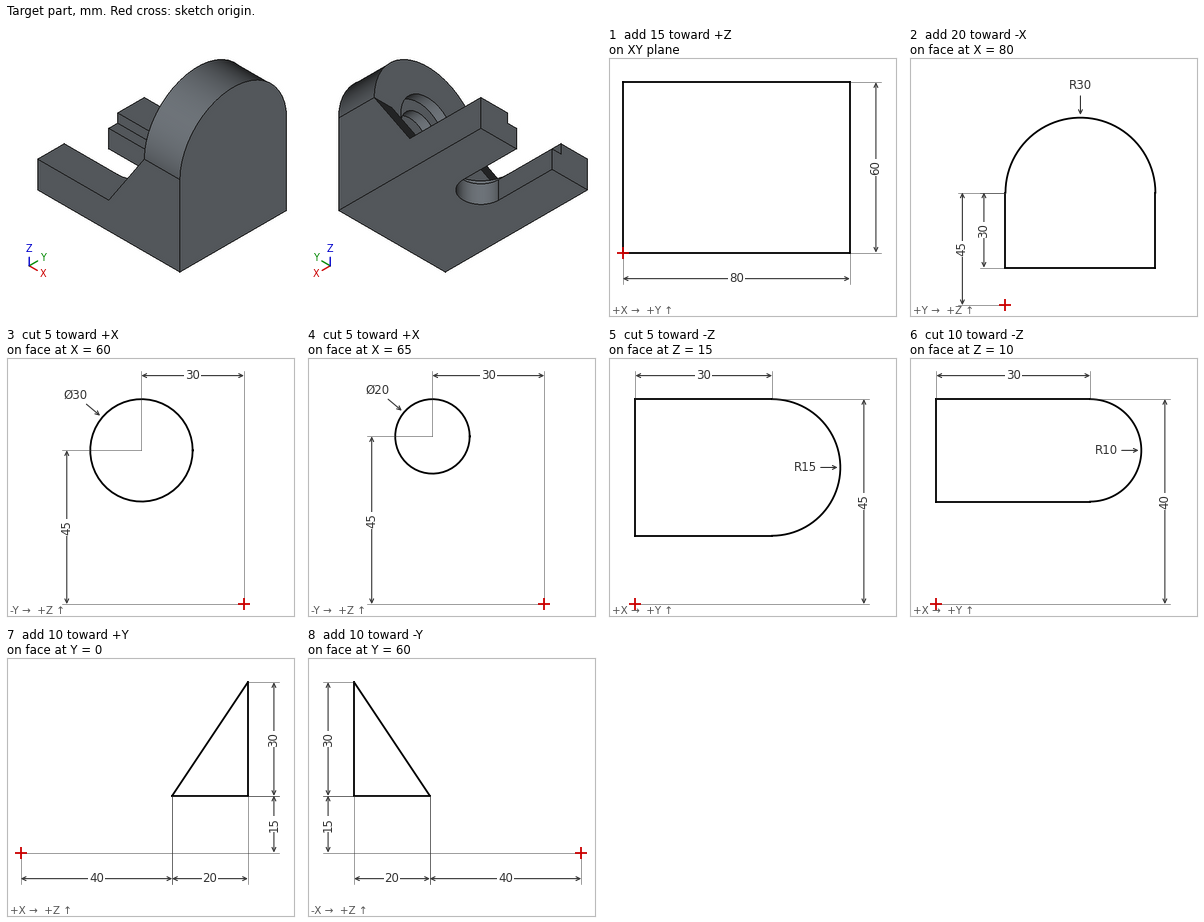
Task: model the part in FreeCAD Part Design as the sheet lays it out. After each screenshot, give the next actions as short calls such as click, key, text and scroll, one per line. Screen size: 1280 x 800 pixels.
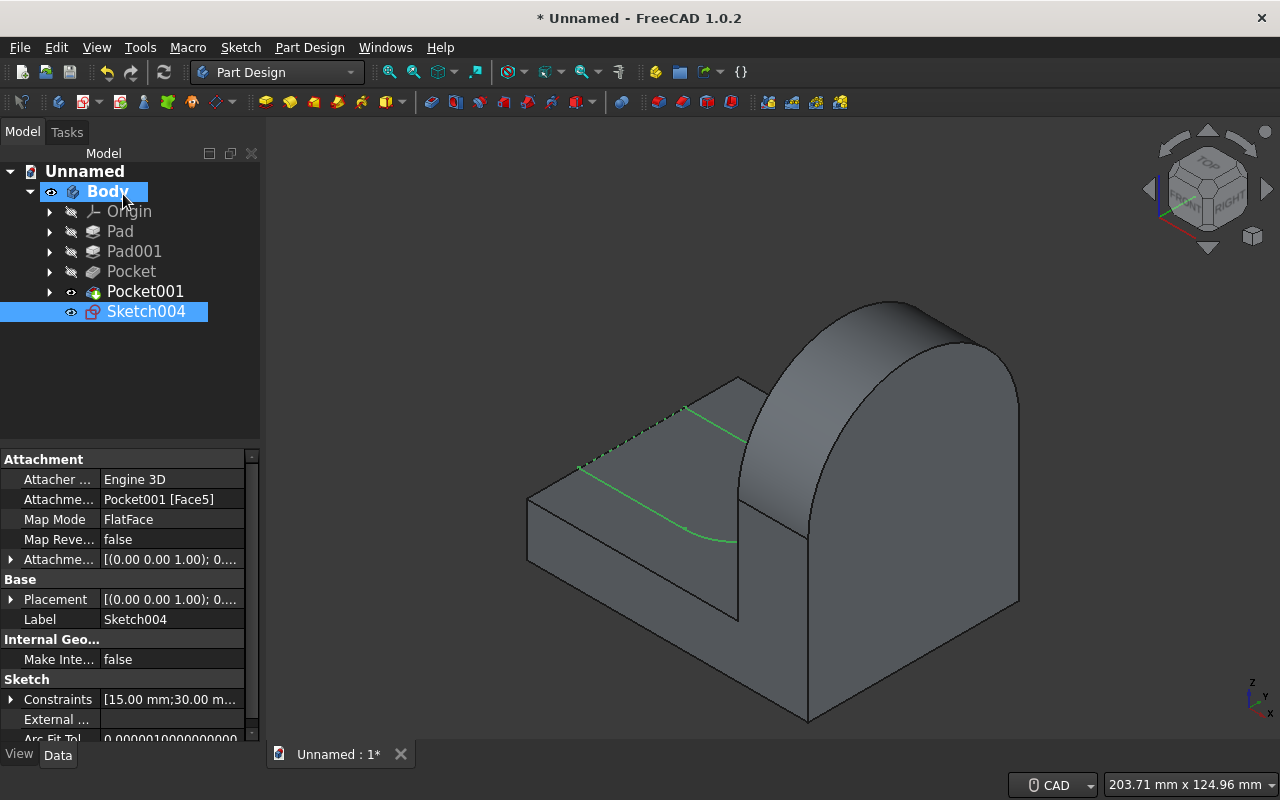
click(432, 102)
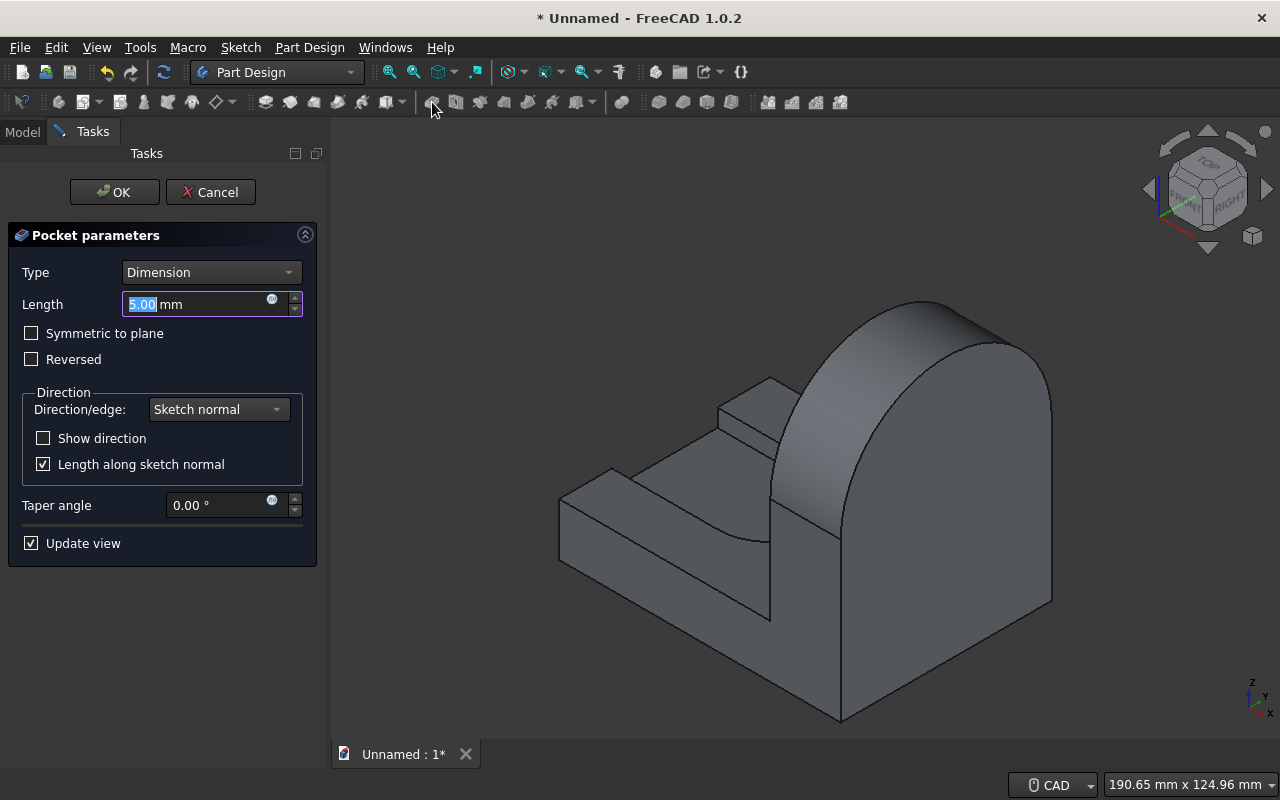
text(5)
key(Tab)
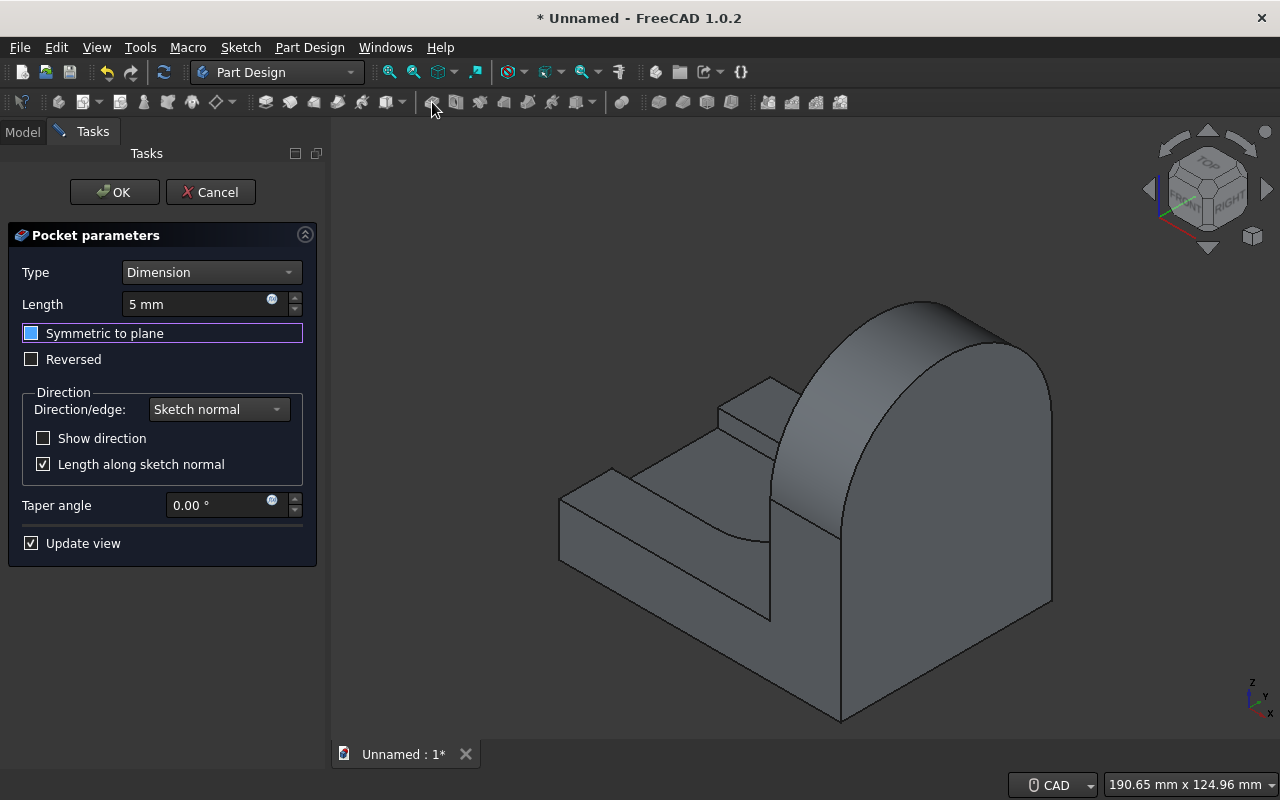
click(115, 192)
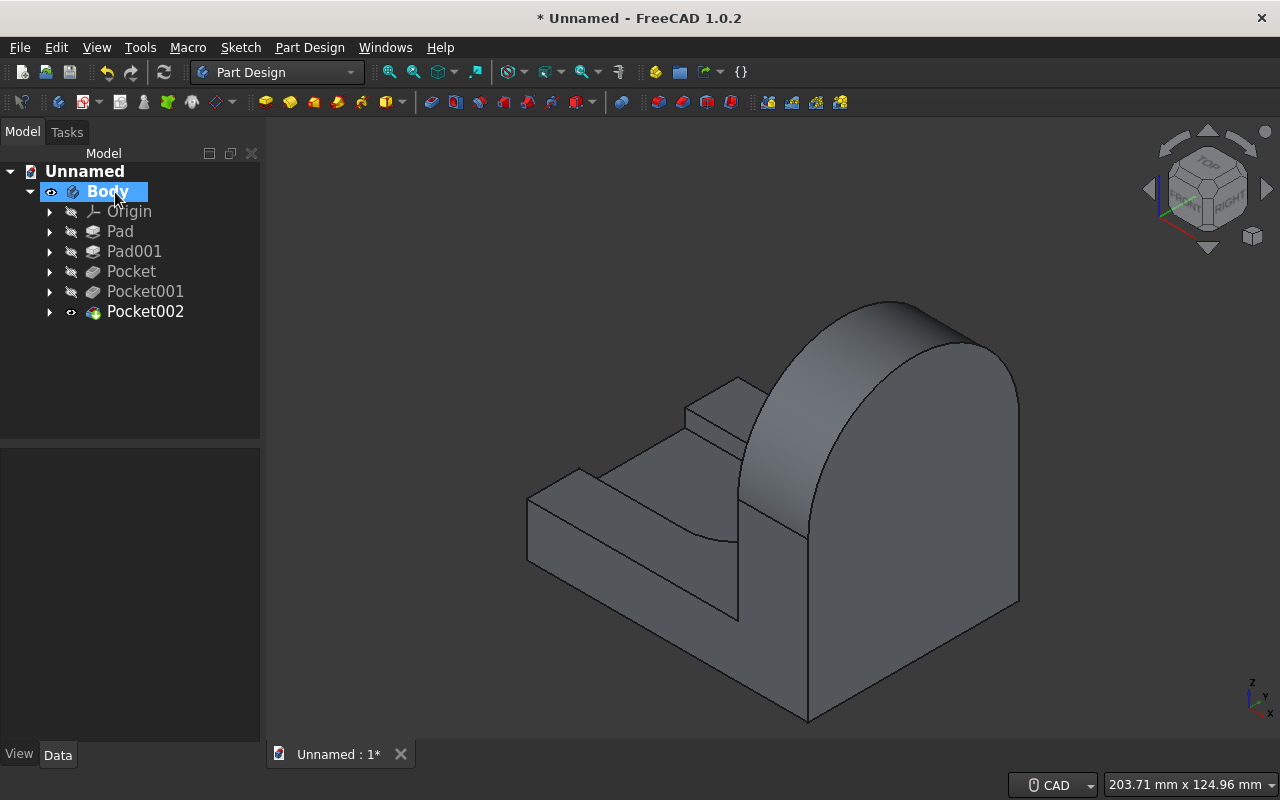
click(711, 503)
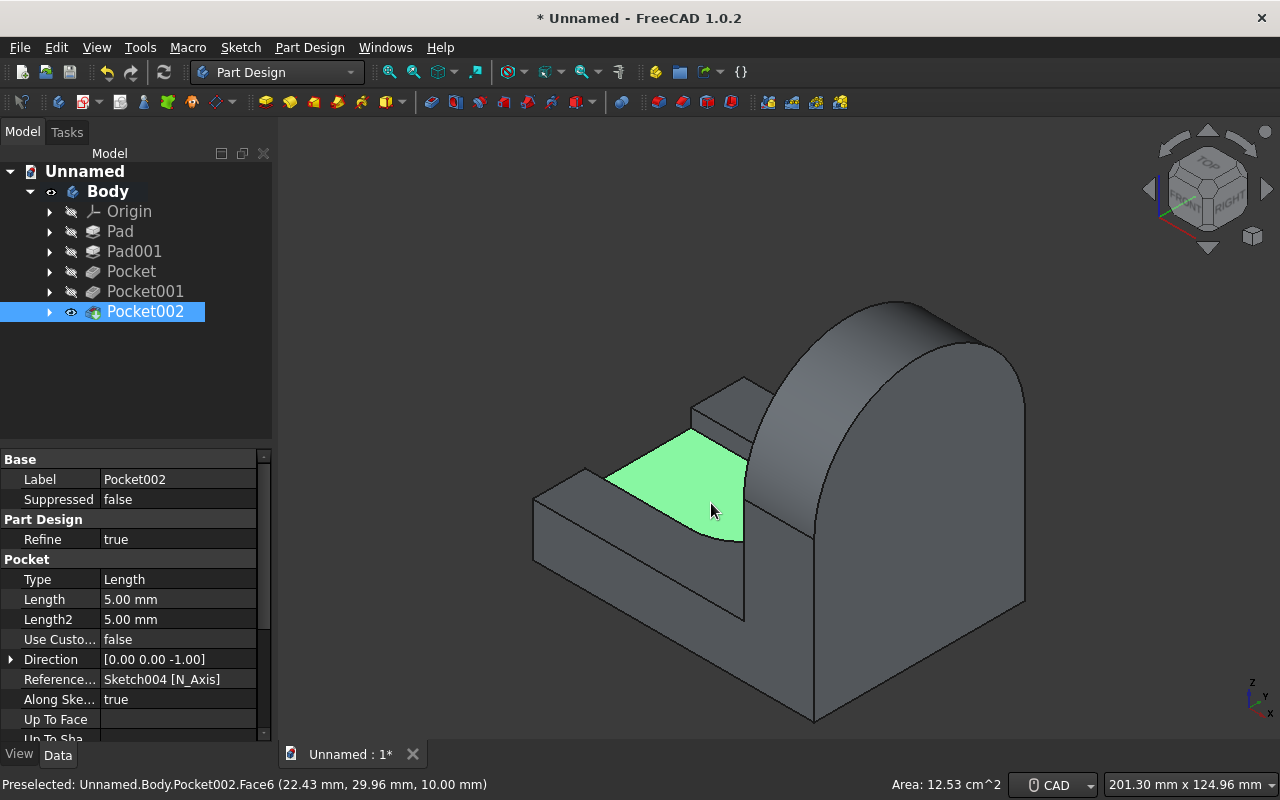
click(84, 102)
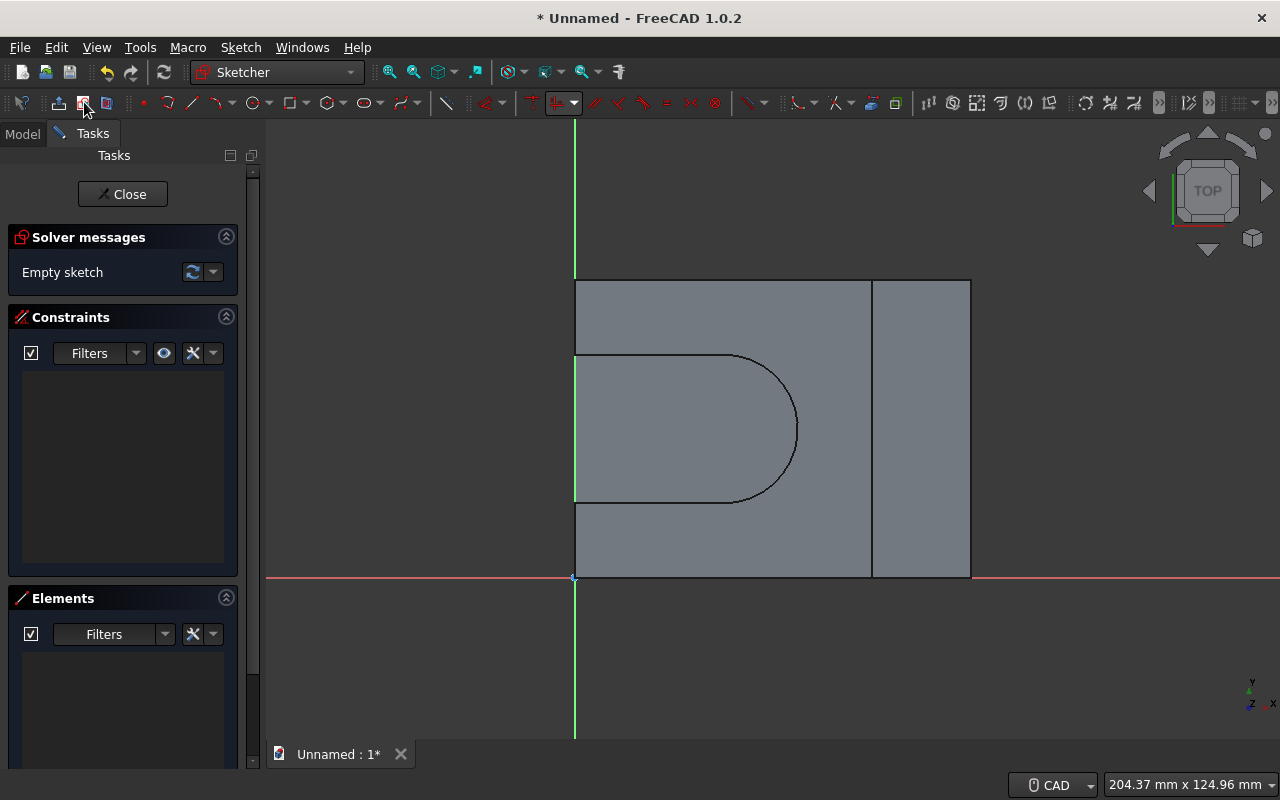
click(108, 104)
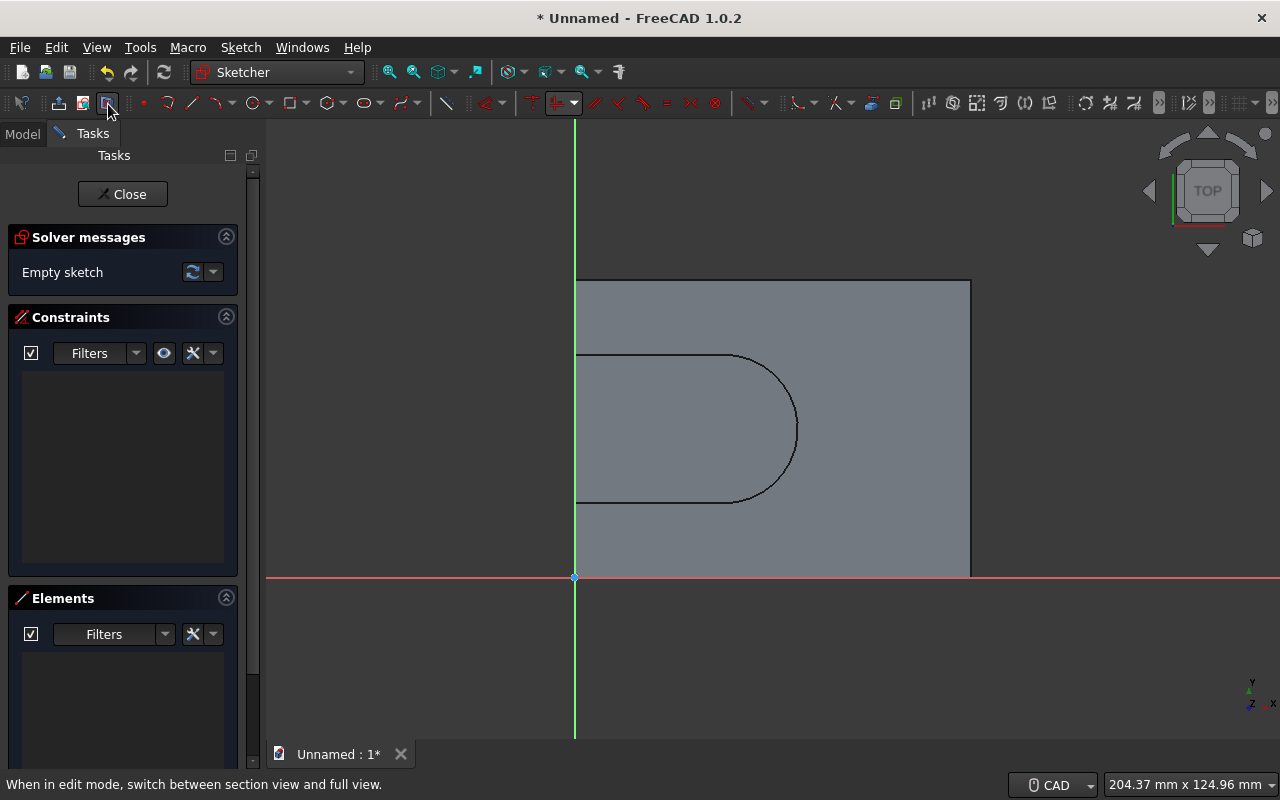
scroll(636, 539, up, 3)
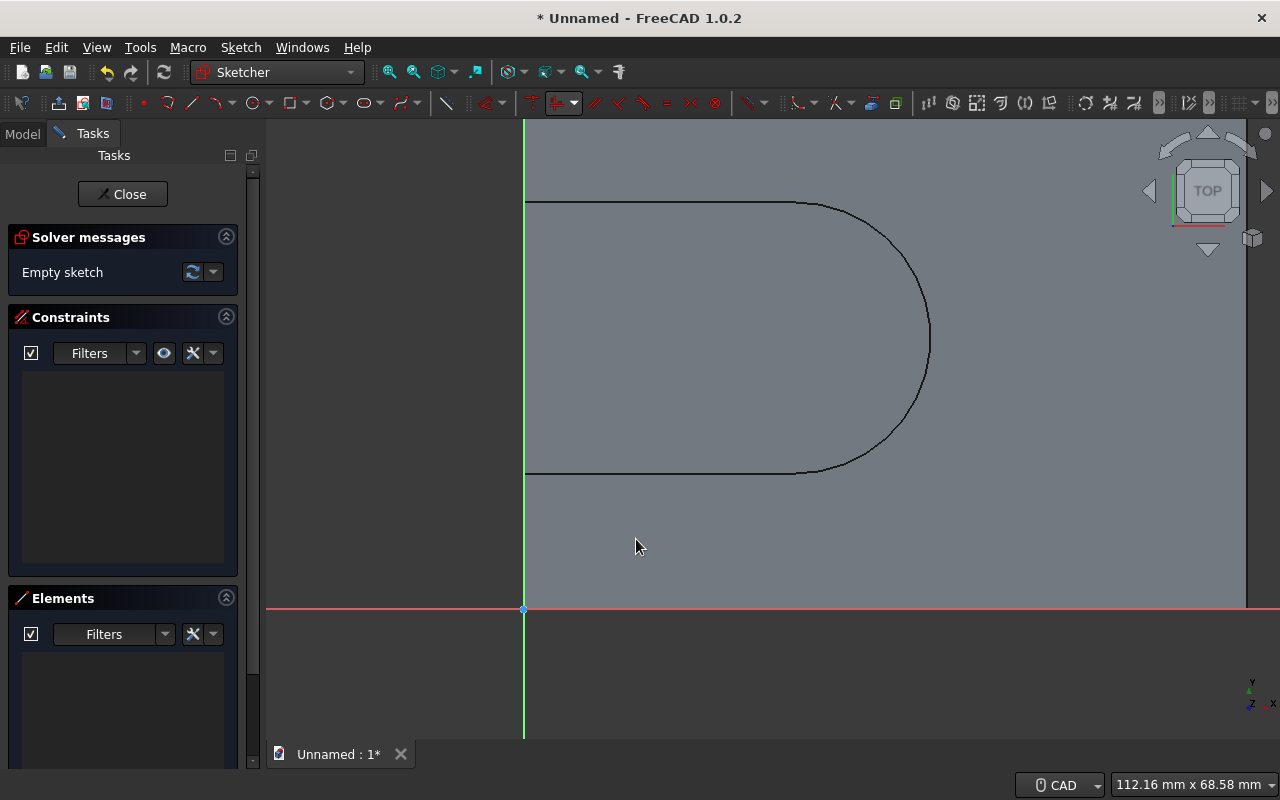
click(168, 104)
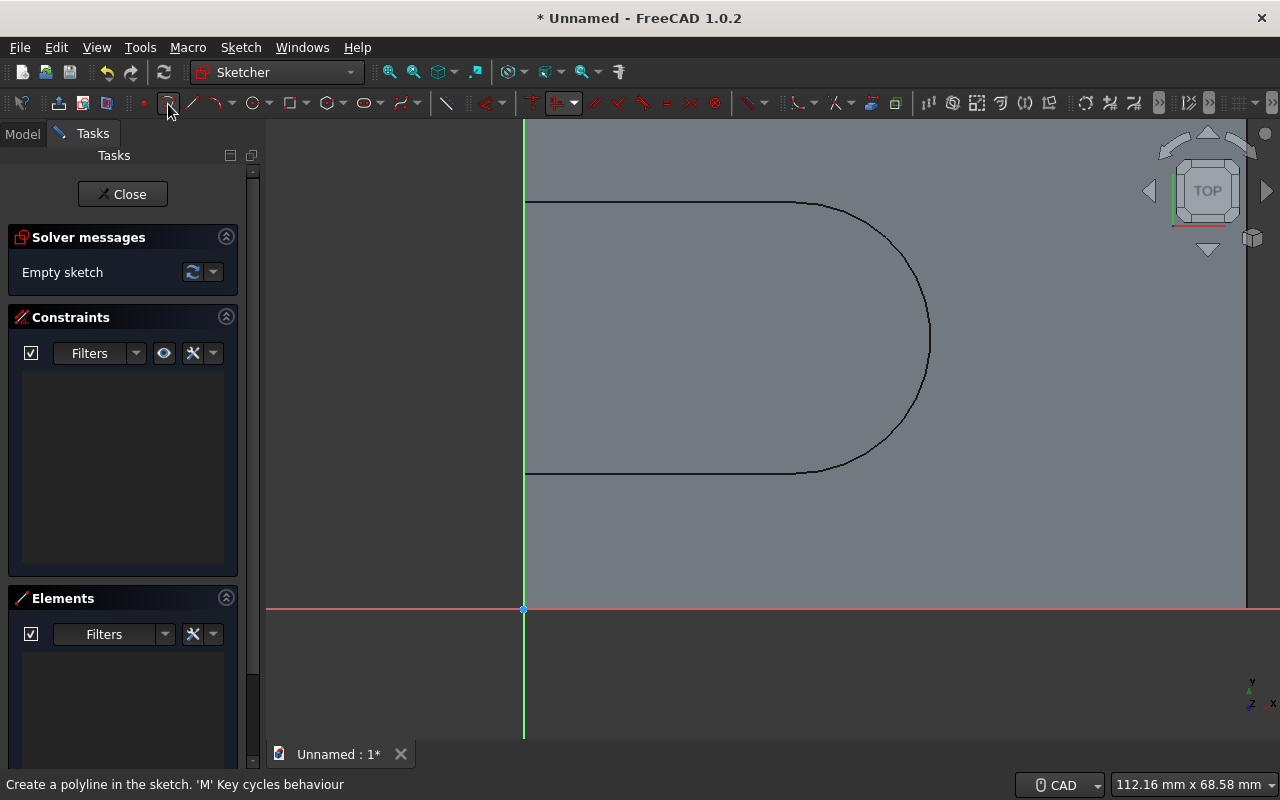
click(795, 248)
click(524, 248)
click(533, 428)
click(795, 428)
right_click(795, 428)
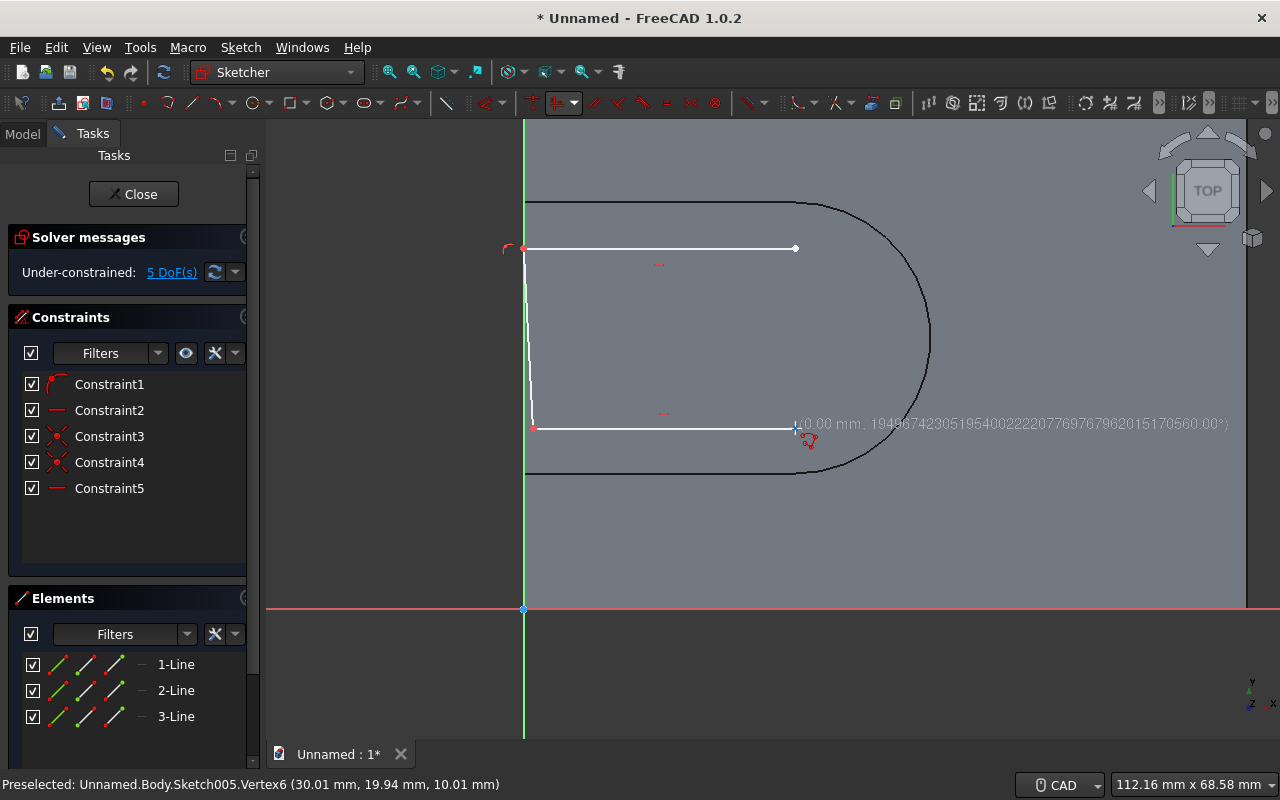
click(216, 104)